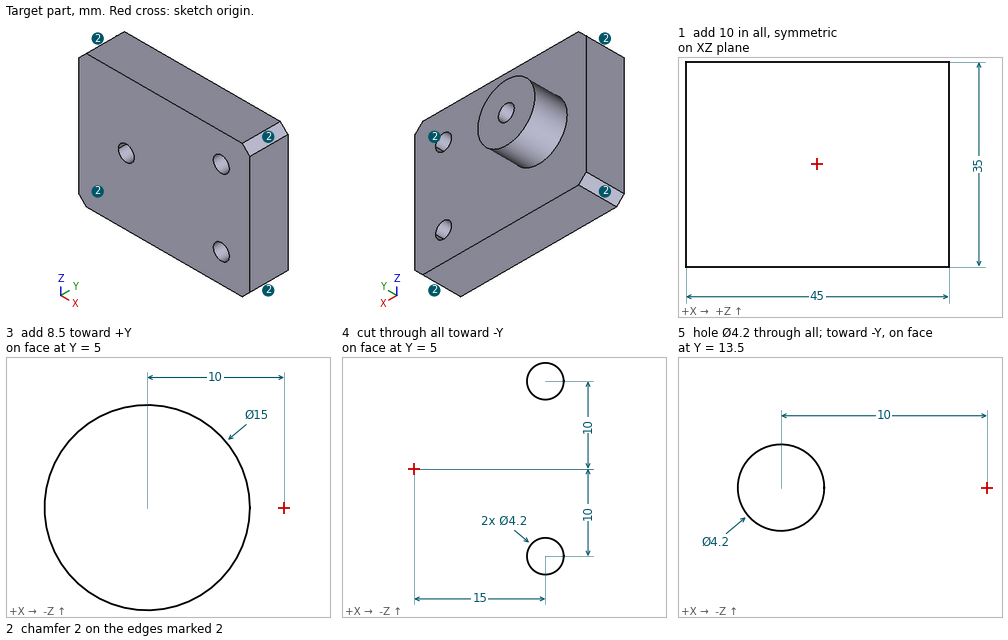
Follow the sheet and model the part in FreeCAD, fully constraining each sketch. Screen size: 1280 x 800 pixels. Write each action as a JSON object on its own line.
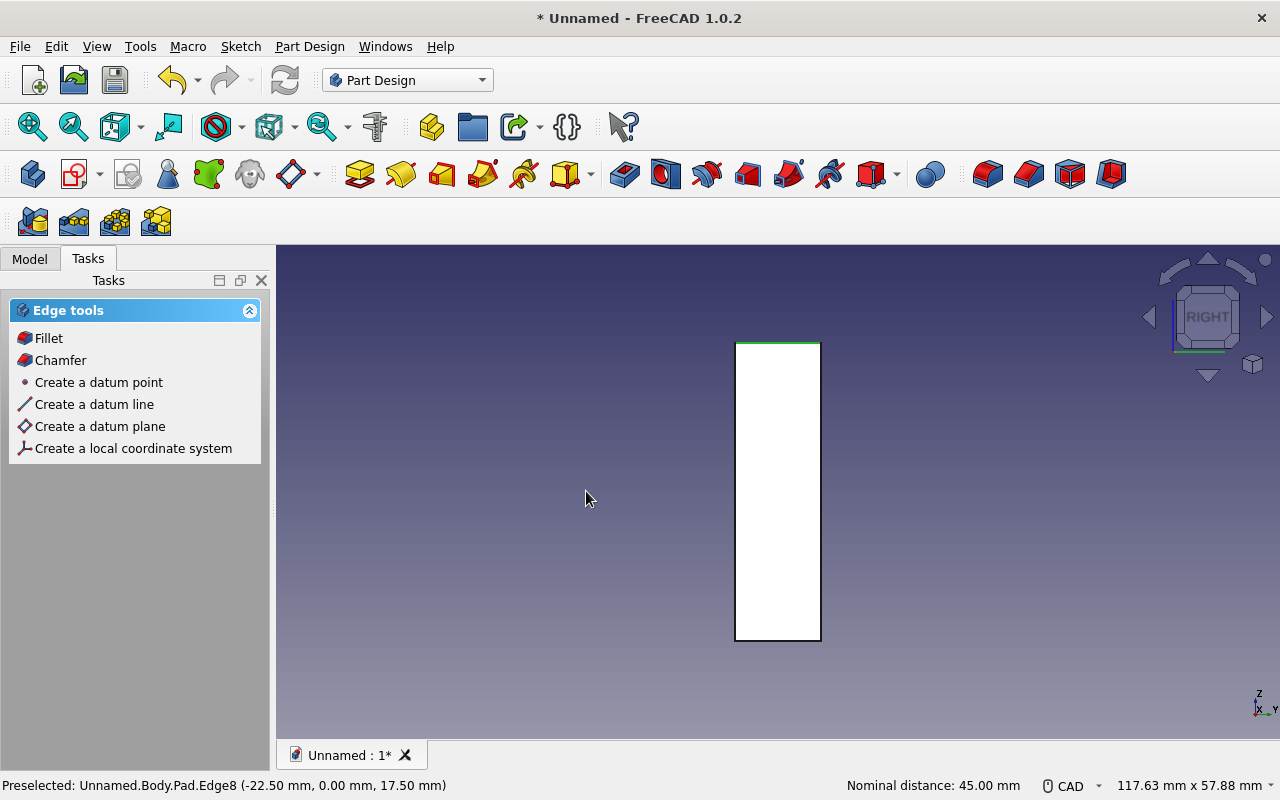
{"action": "left_click", "coordinate": [778, 640], "text": "ctrl"}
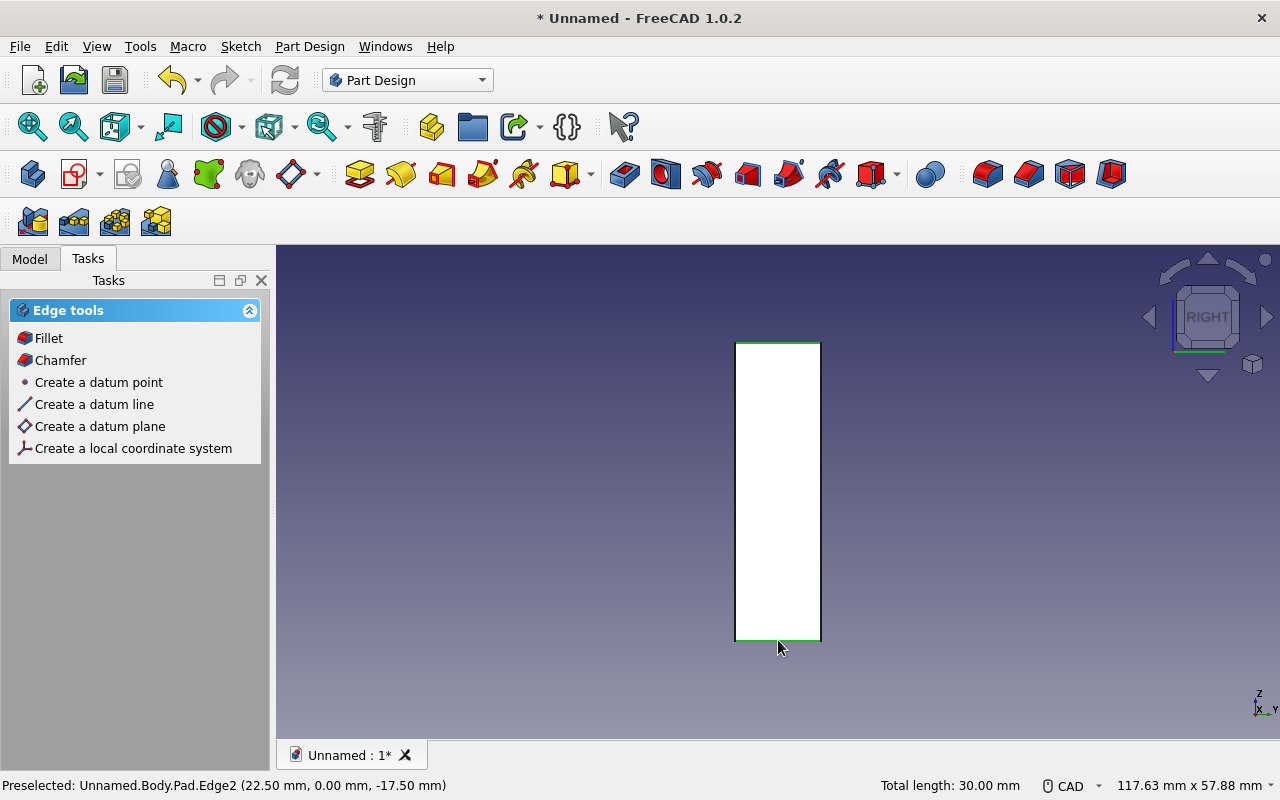
{"action": "key", "text": "5"}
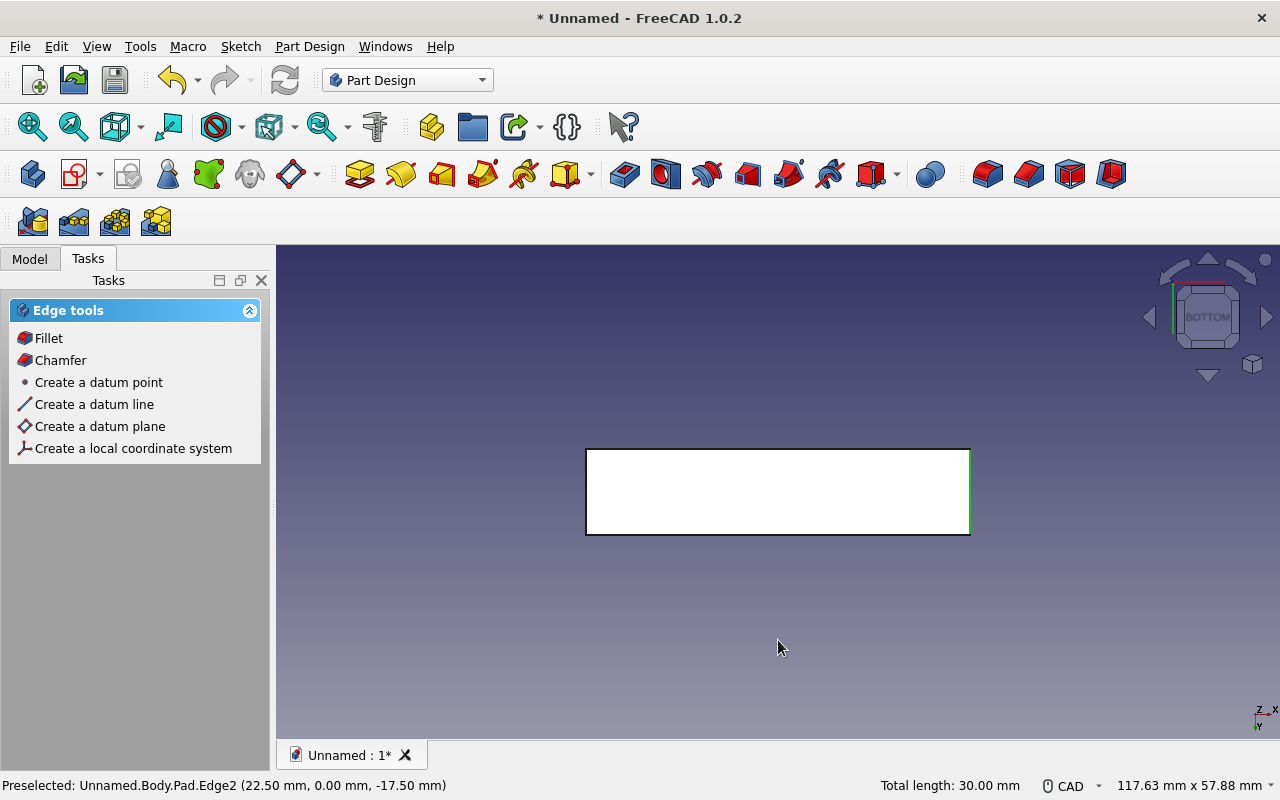
{"action": "left_click", "coordinate": [33, 128]}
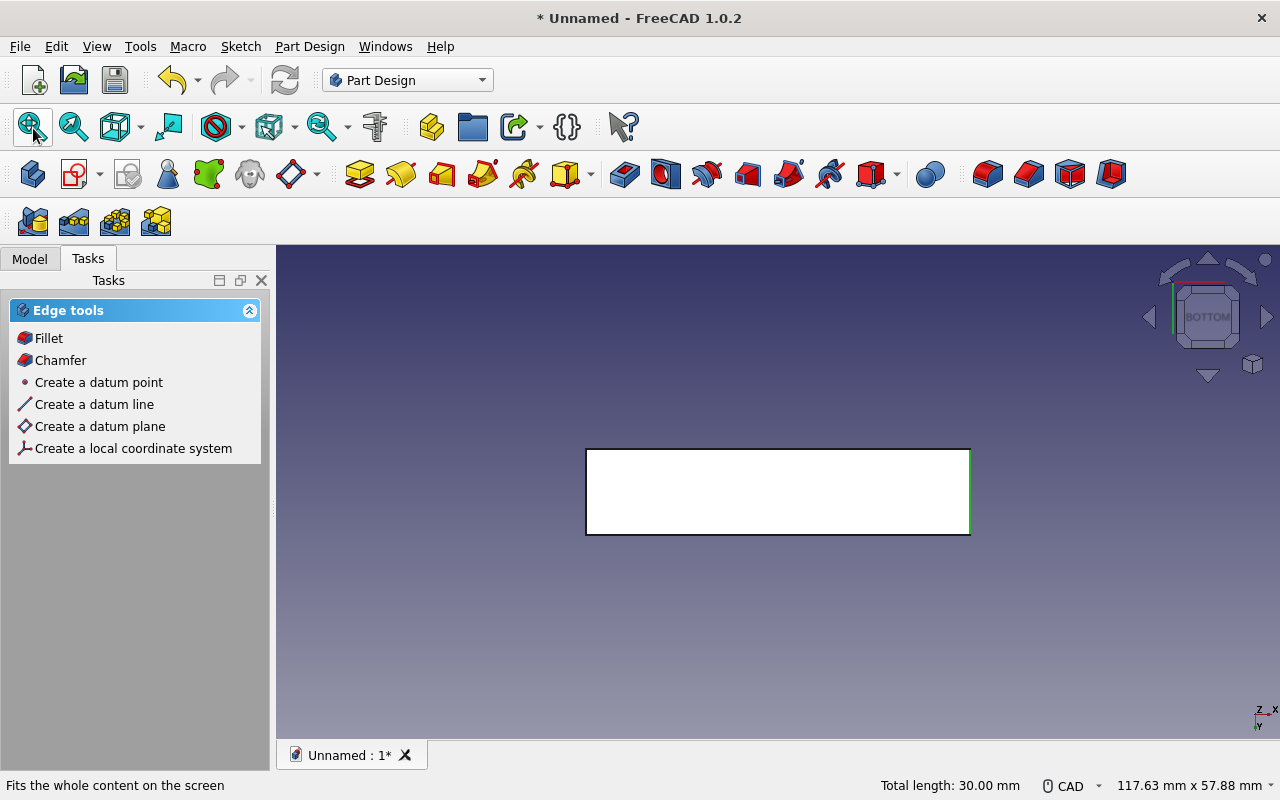
{"action": "left_click", "coordinate": [586, 491], "text": "ctrl"}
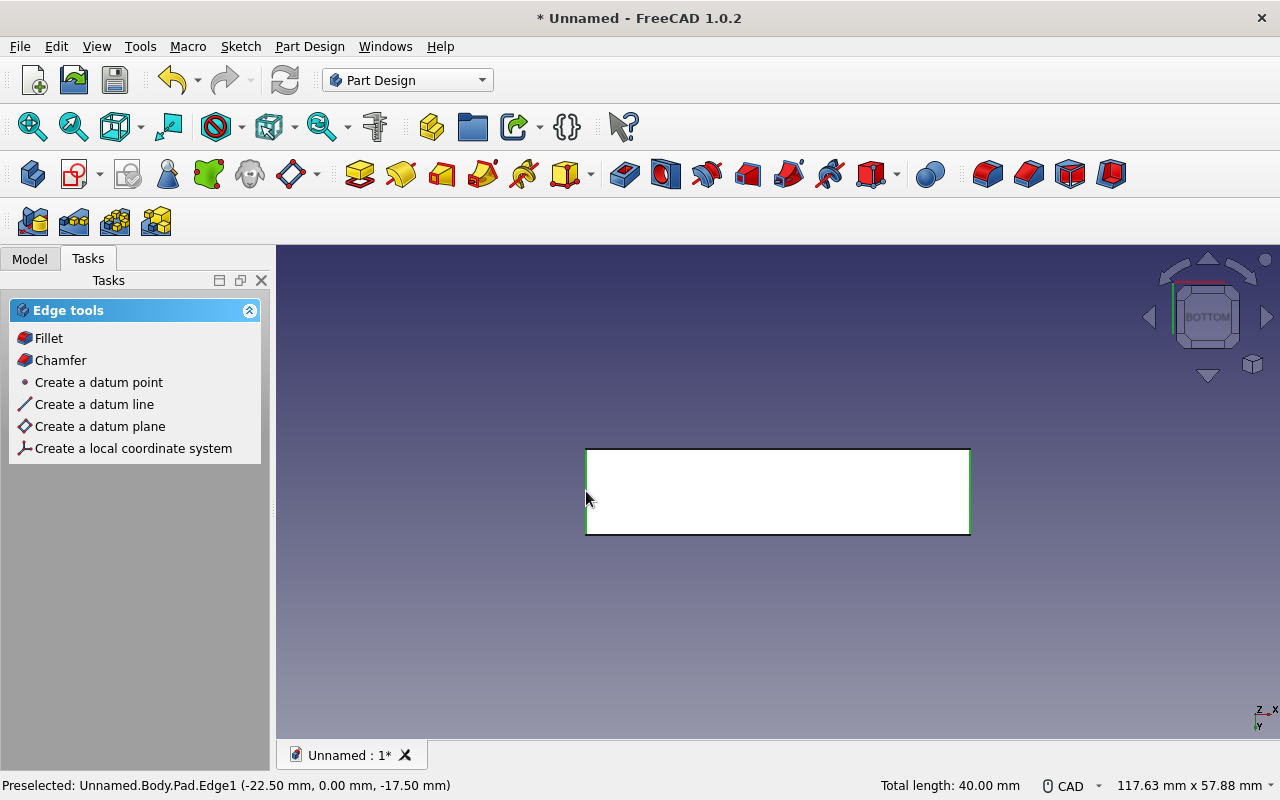
{"action": "left_click", "coordinate": [1029, 174]}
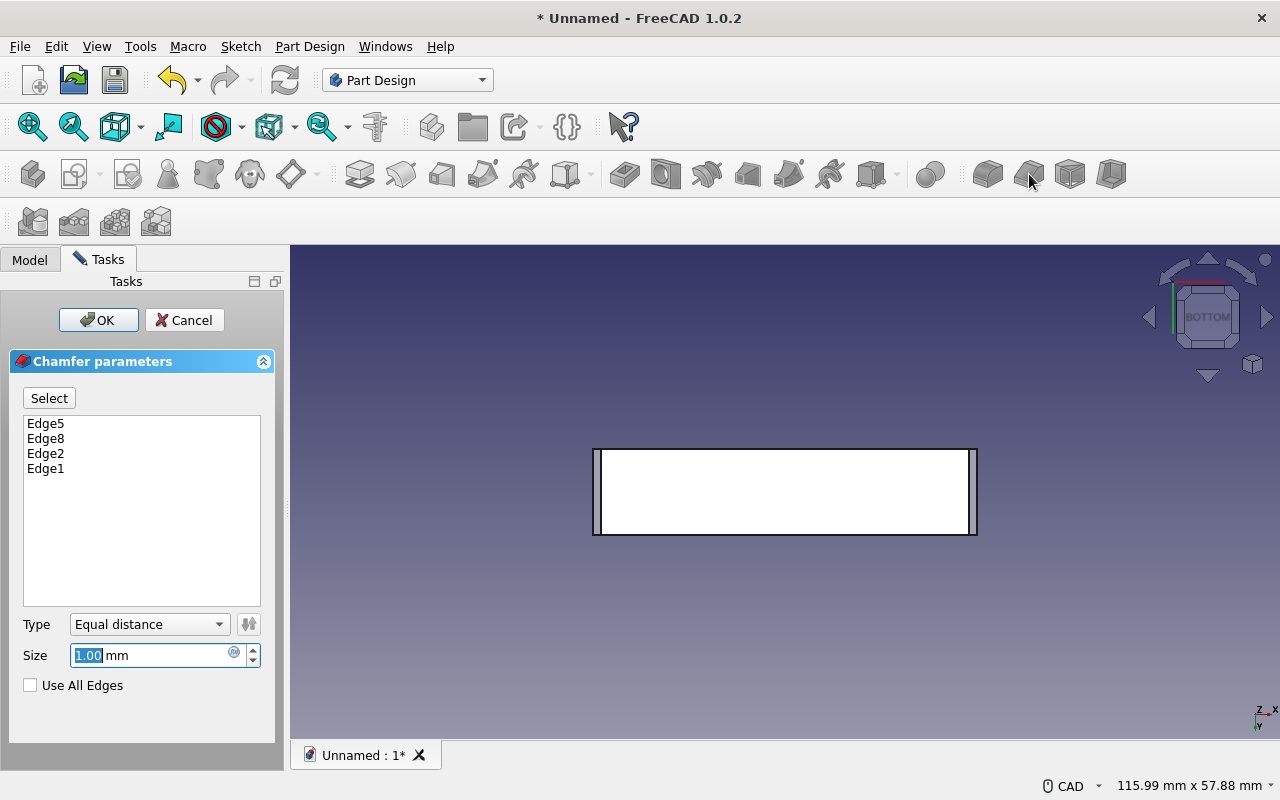
{"action": "type", "text": "2"}
{"action": "key", "text": "Tab"}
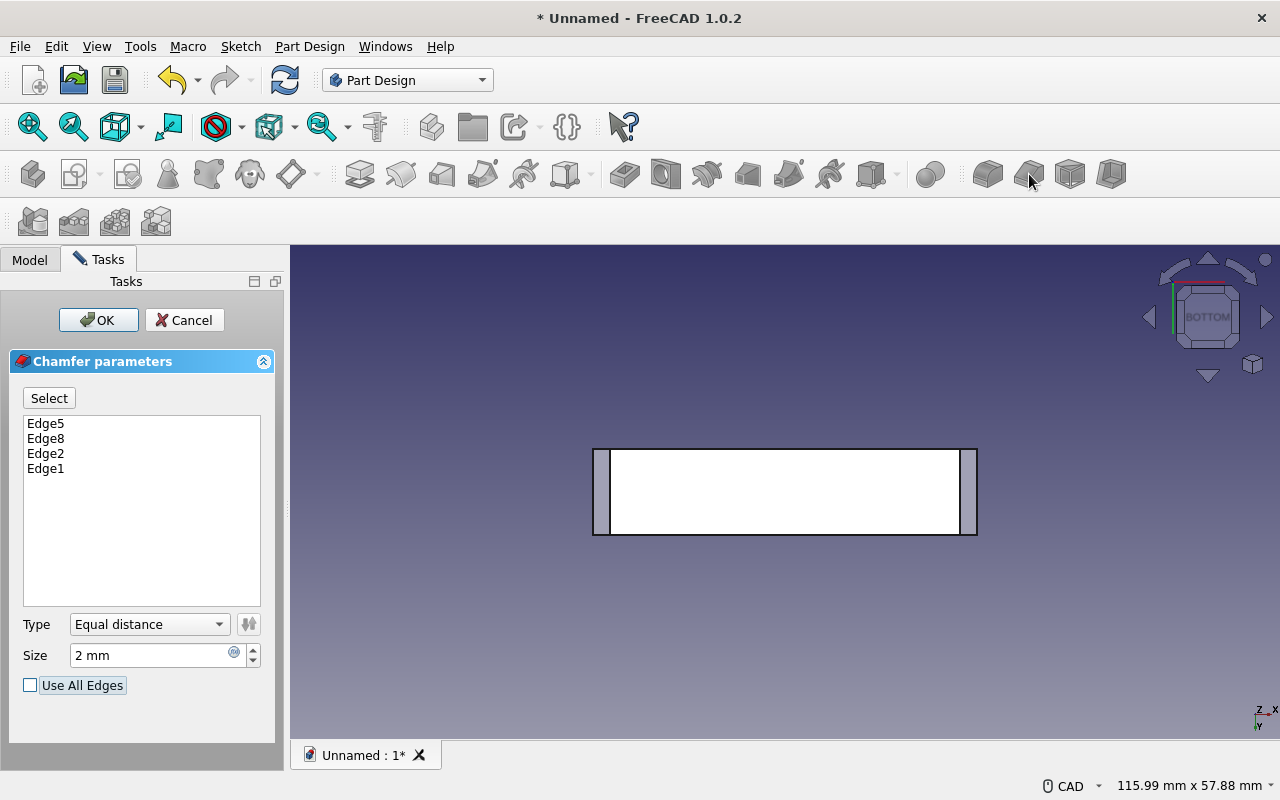
{"action": "left_click", "coordinate": [99, 320]}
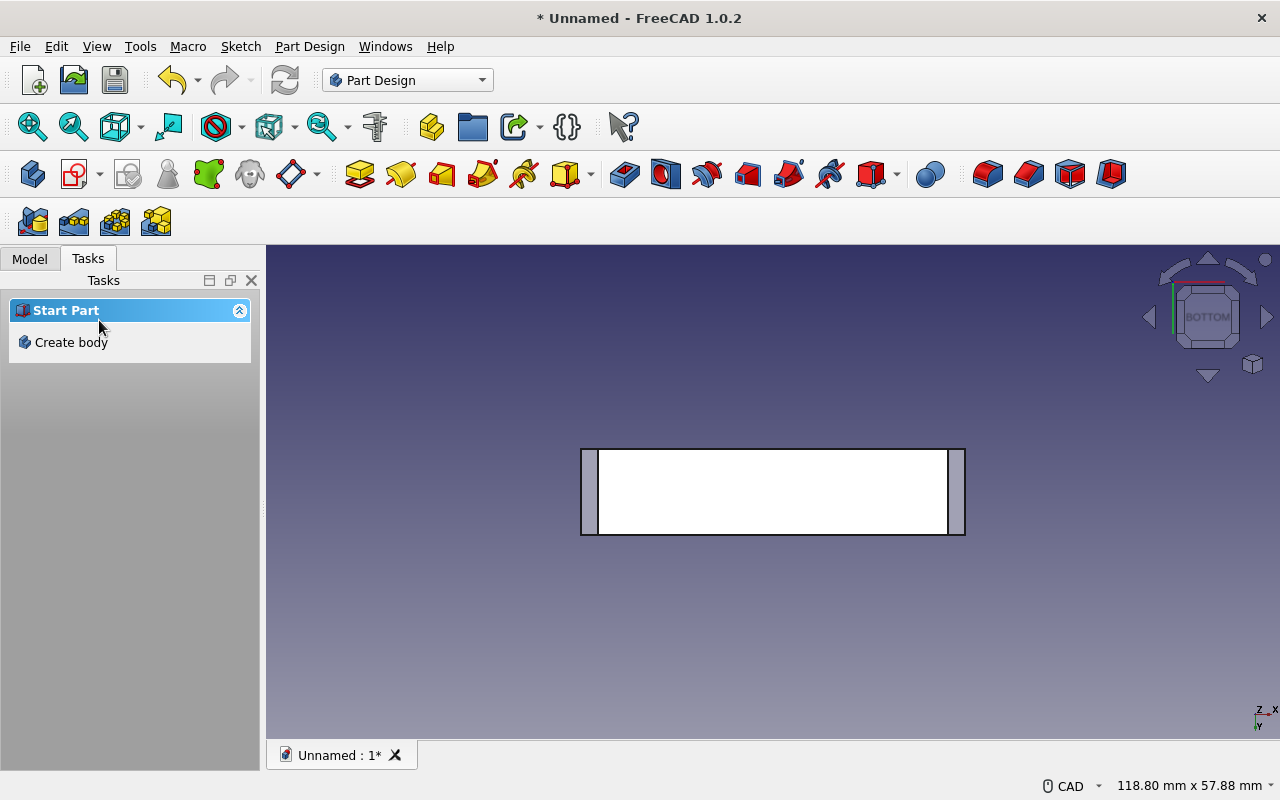
{"action": "key", "text": "v f"}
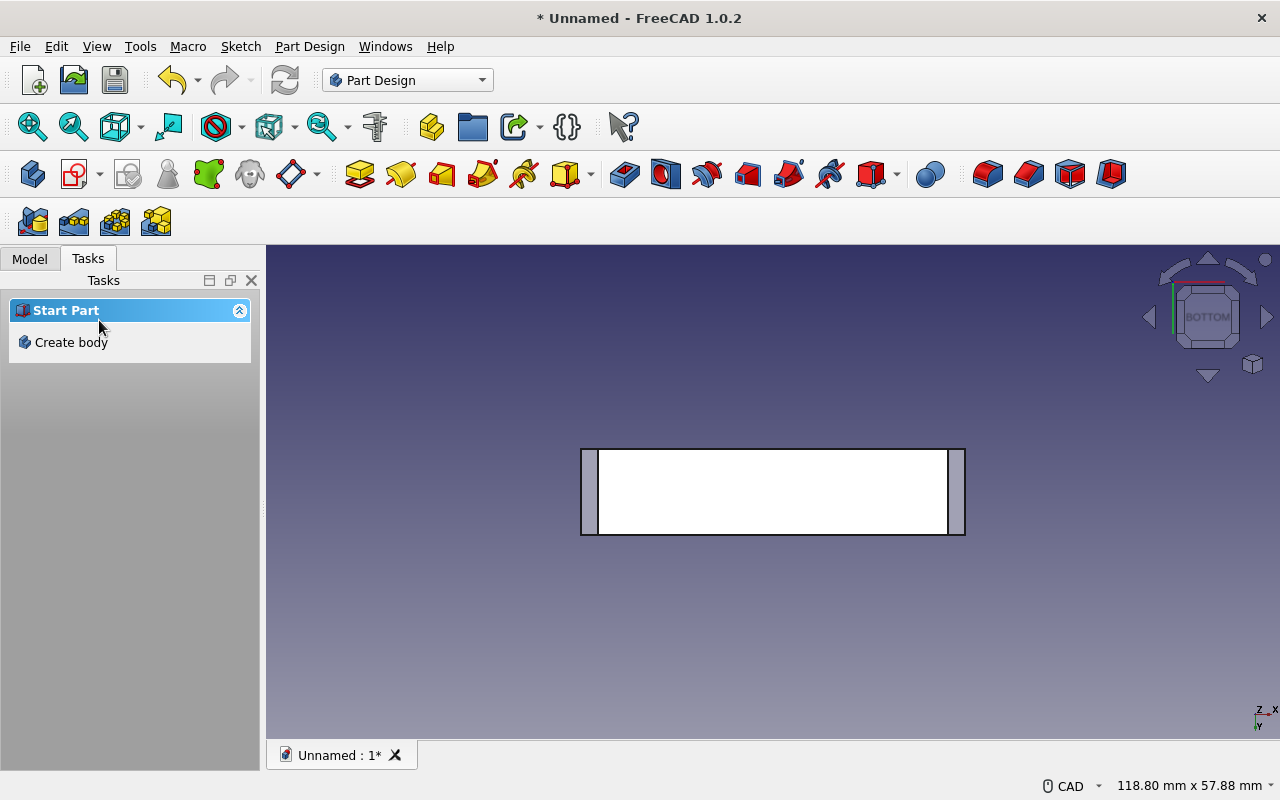
{"action": "key", "text": "4"}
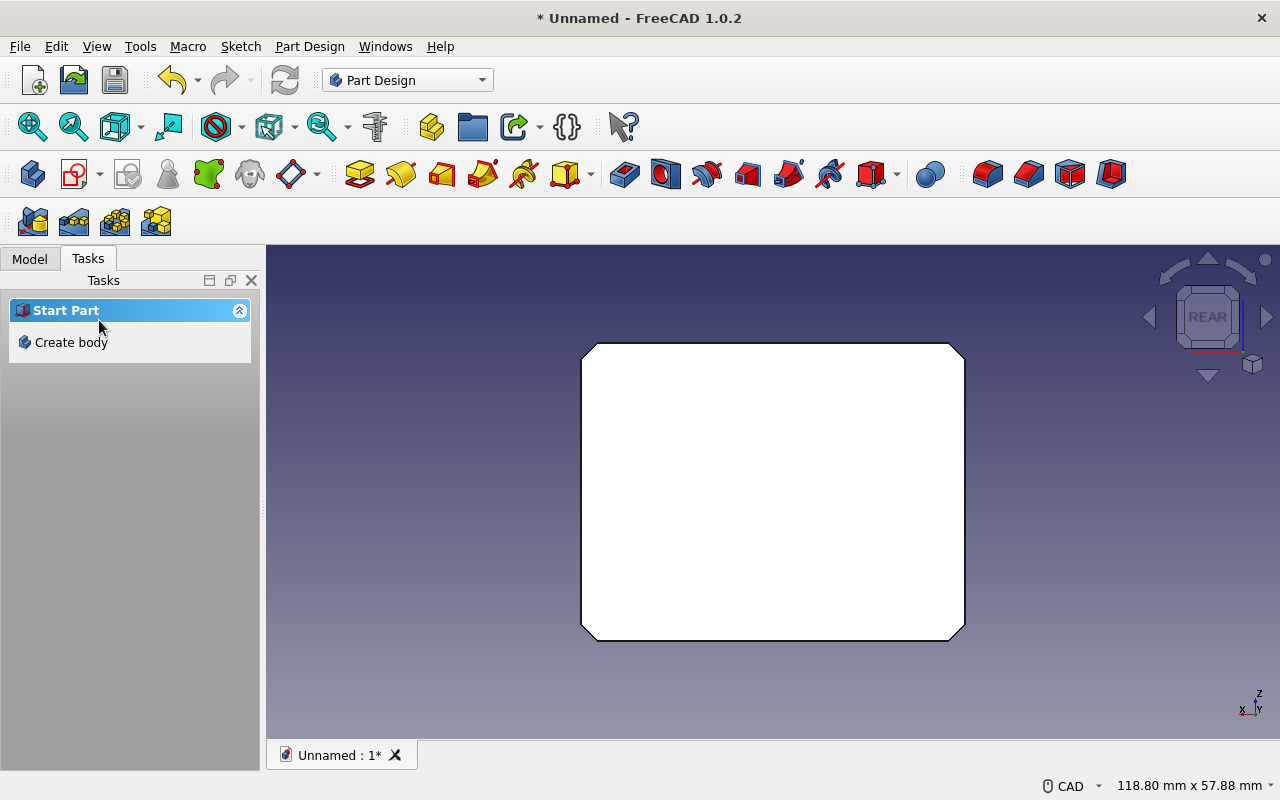
{"action": "left_click", "coordinate": [773, 491]}